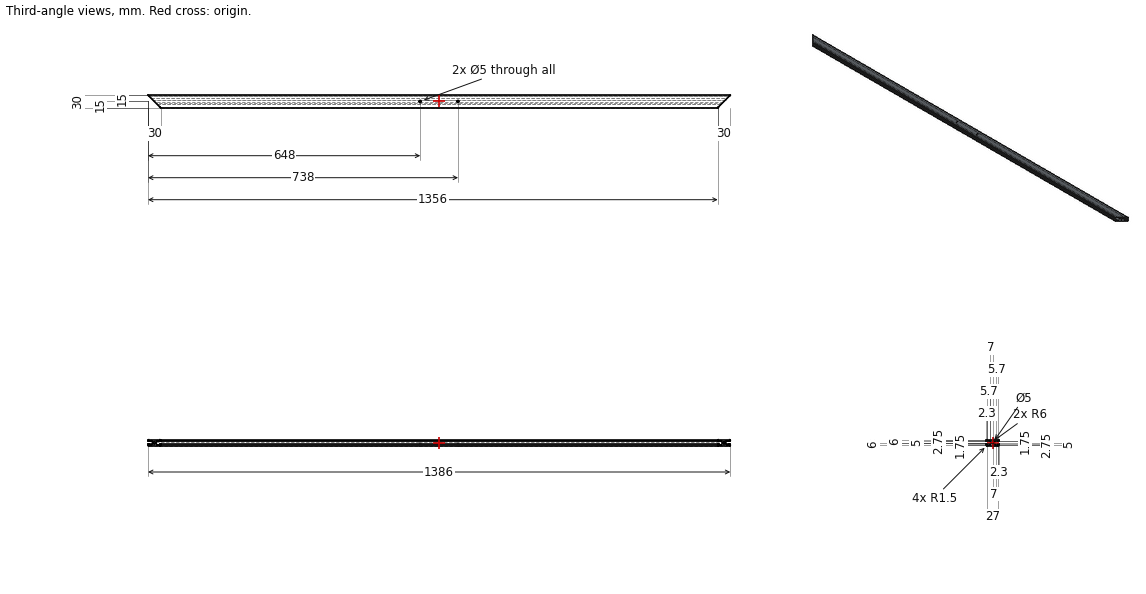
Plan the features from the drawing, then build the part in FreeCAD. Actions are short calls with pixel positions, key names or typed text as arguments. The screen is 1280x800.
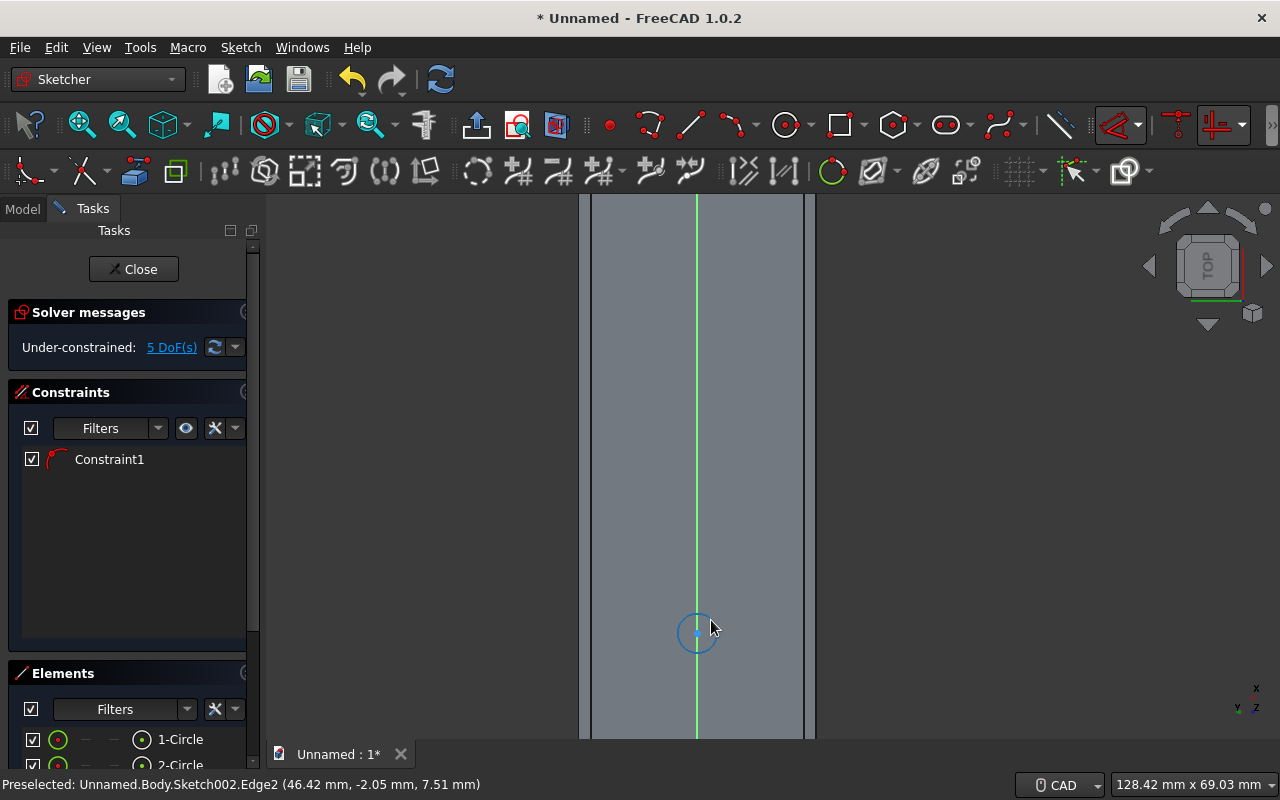
click(711, 619)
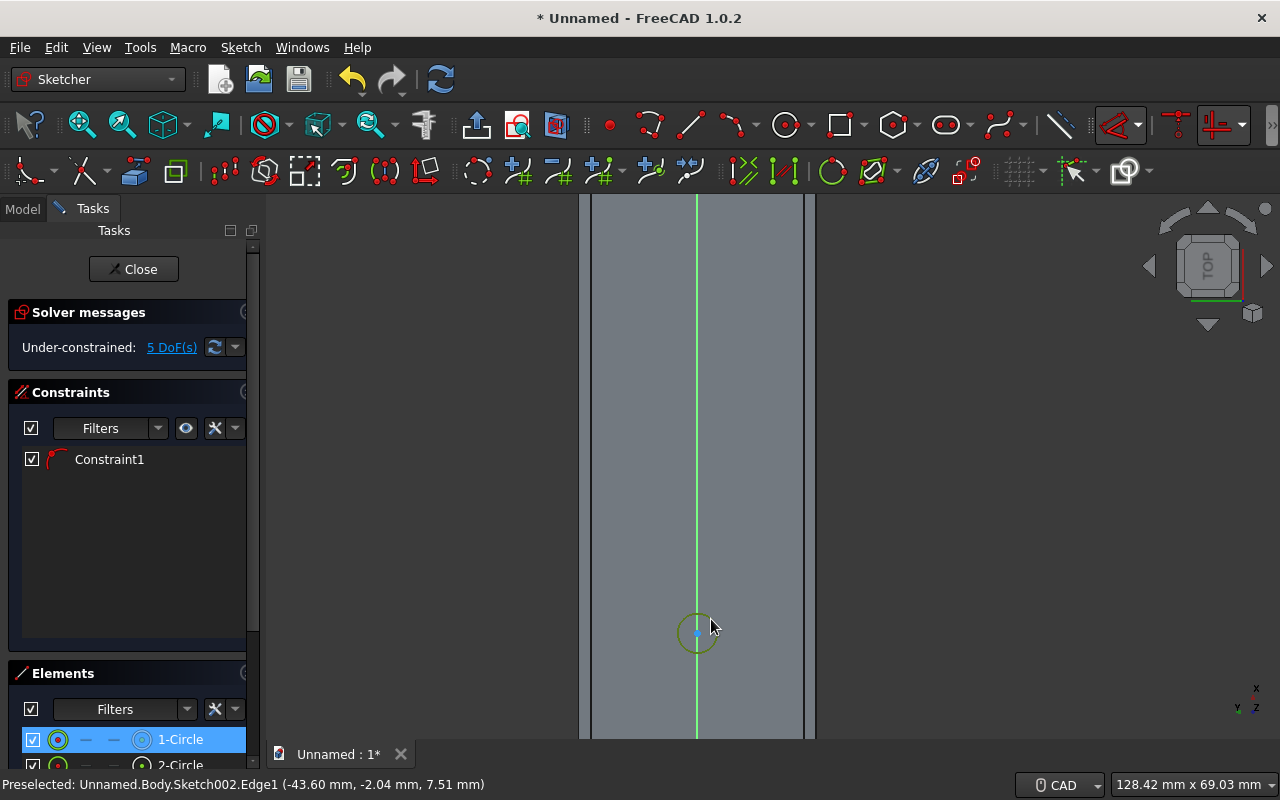
scroll(710, 621, down, 4)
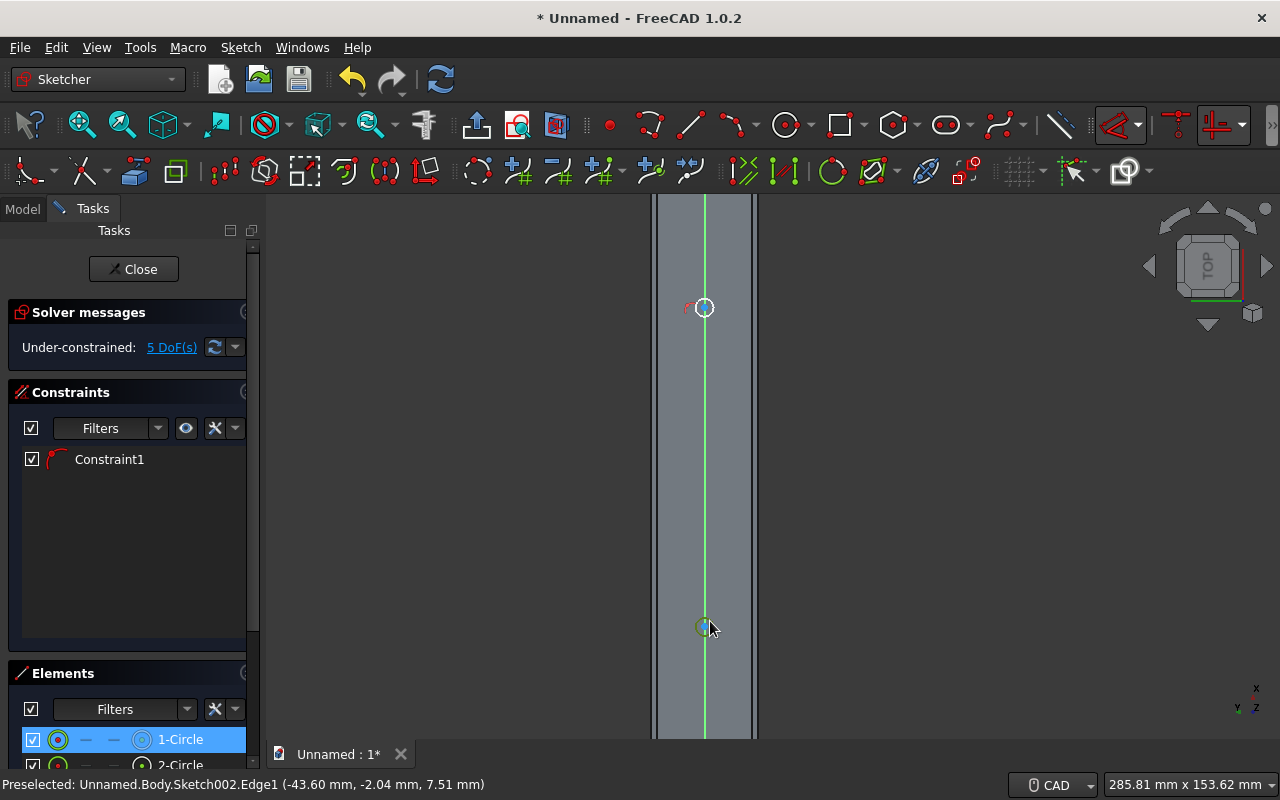
scroll(711, 301, up, 4)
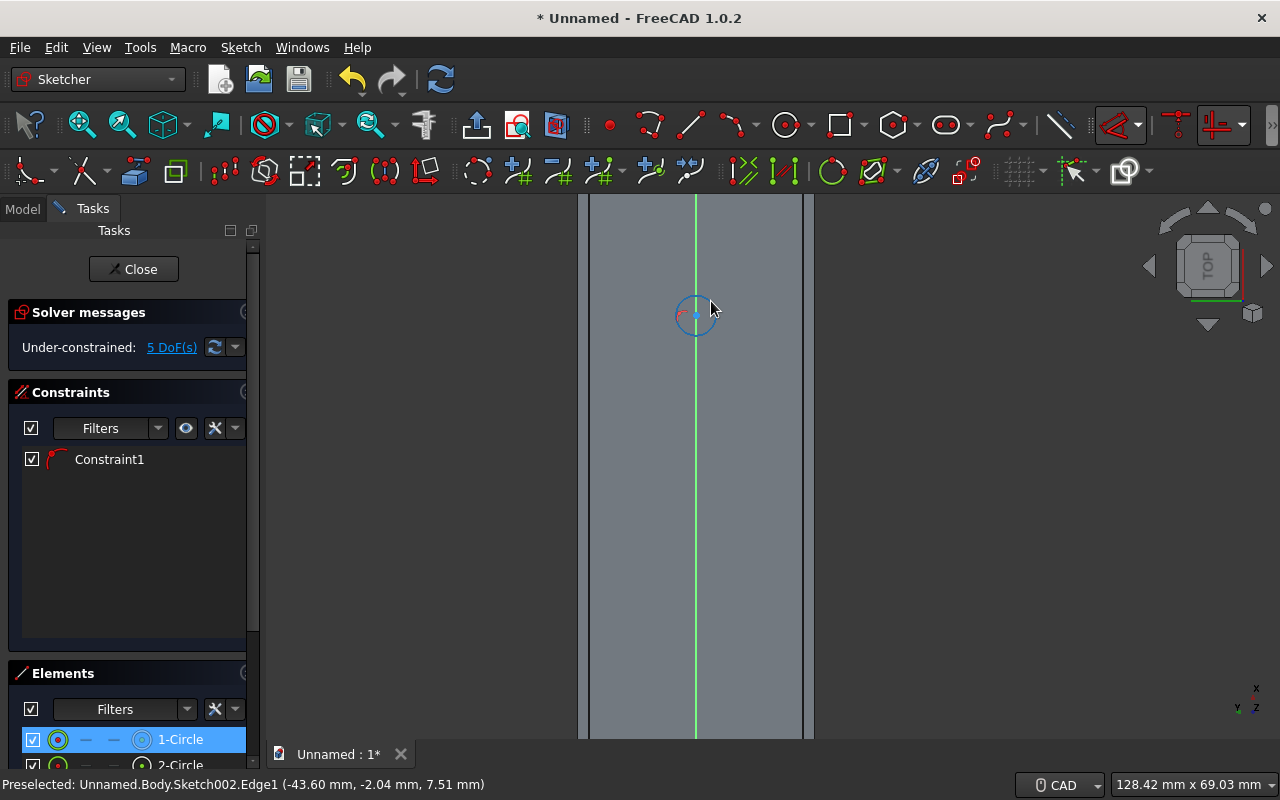
click(710, 301)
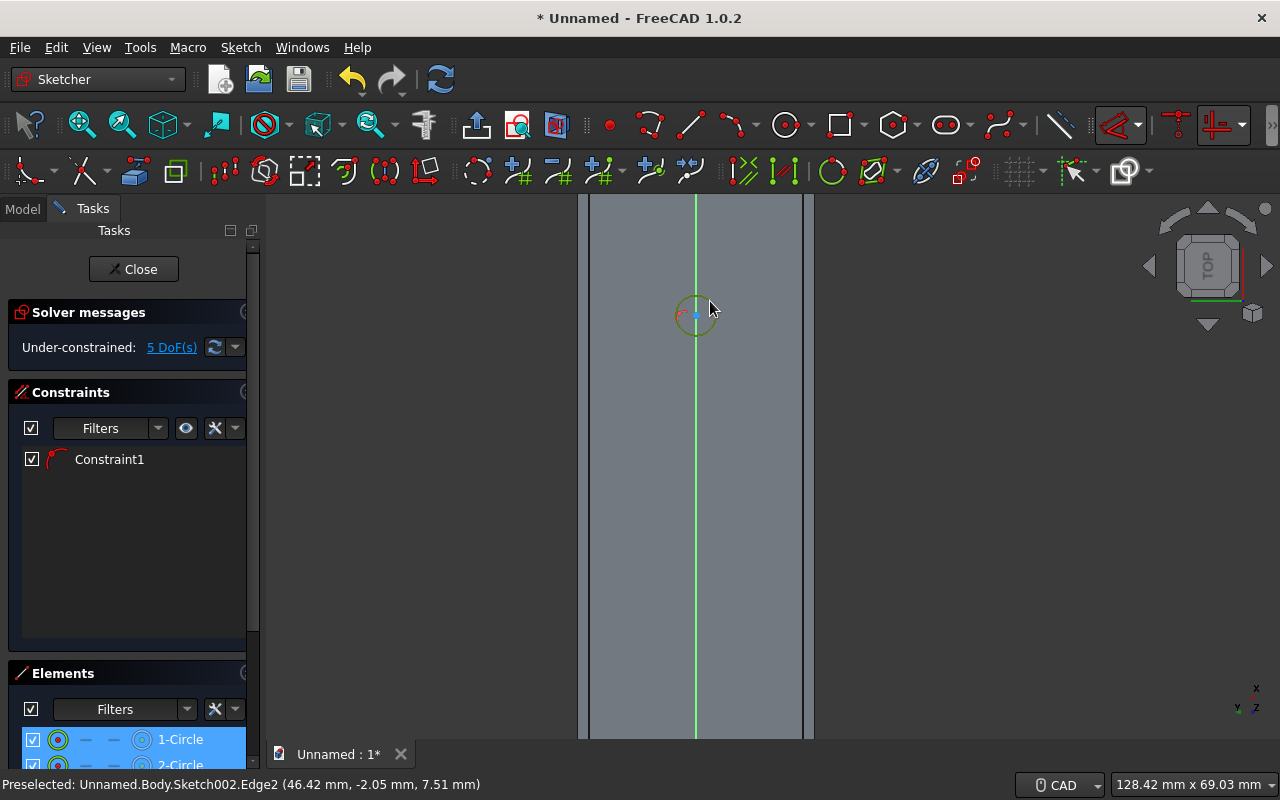
key(e)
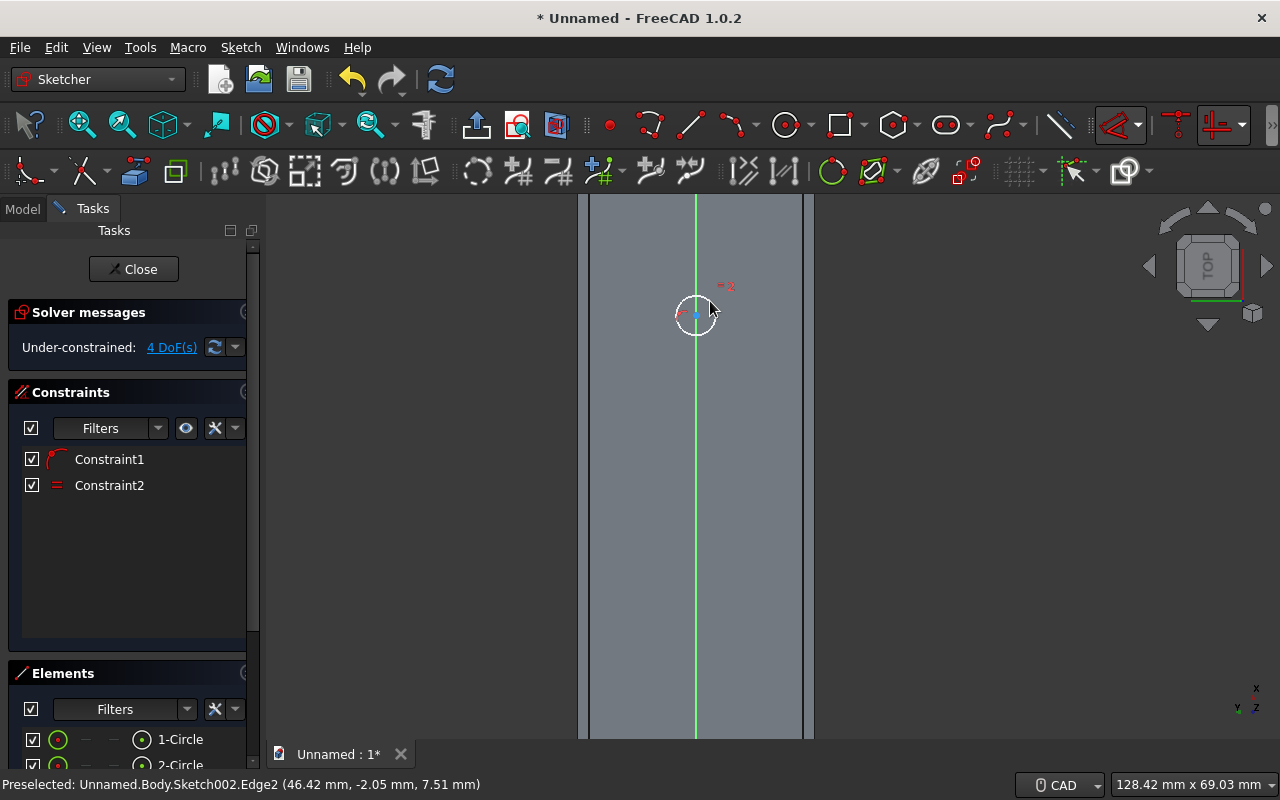
scroll(711, 300, down, 4)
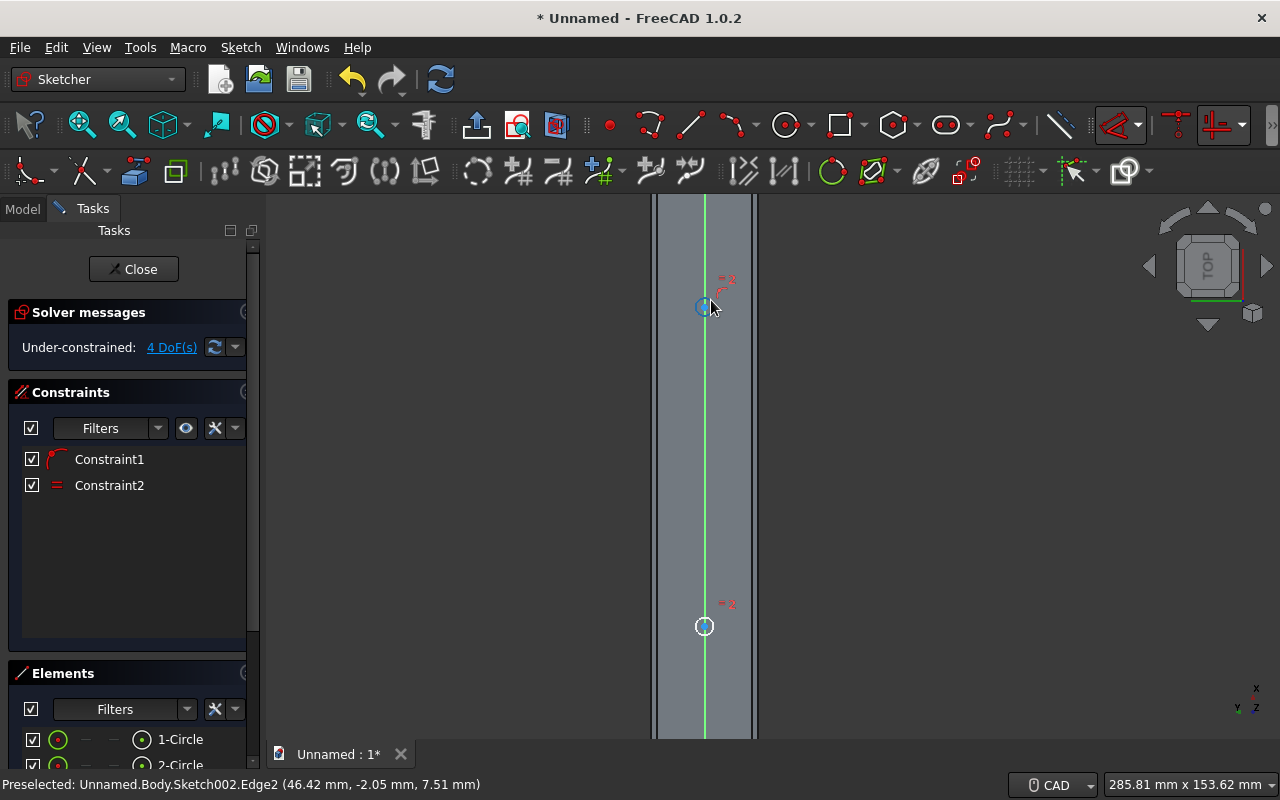
click(705, 626)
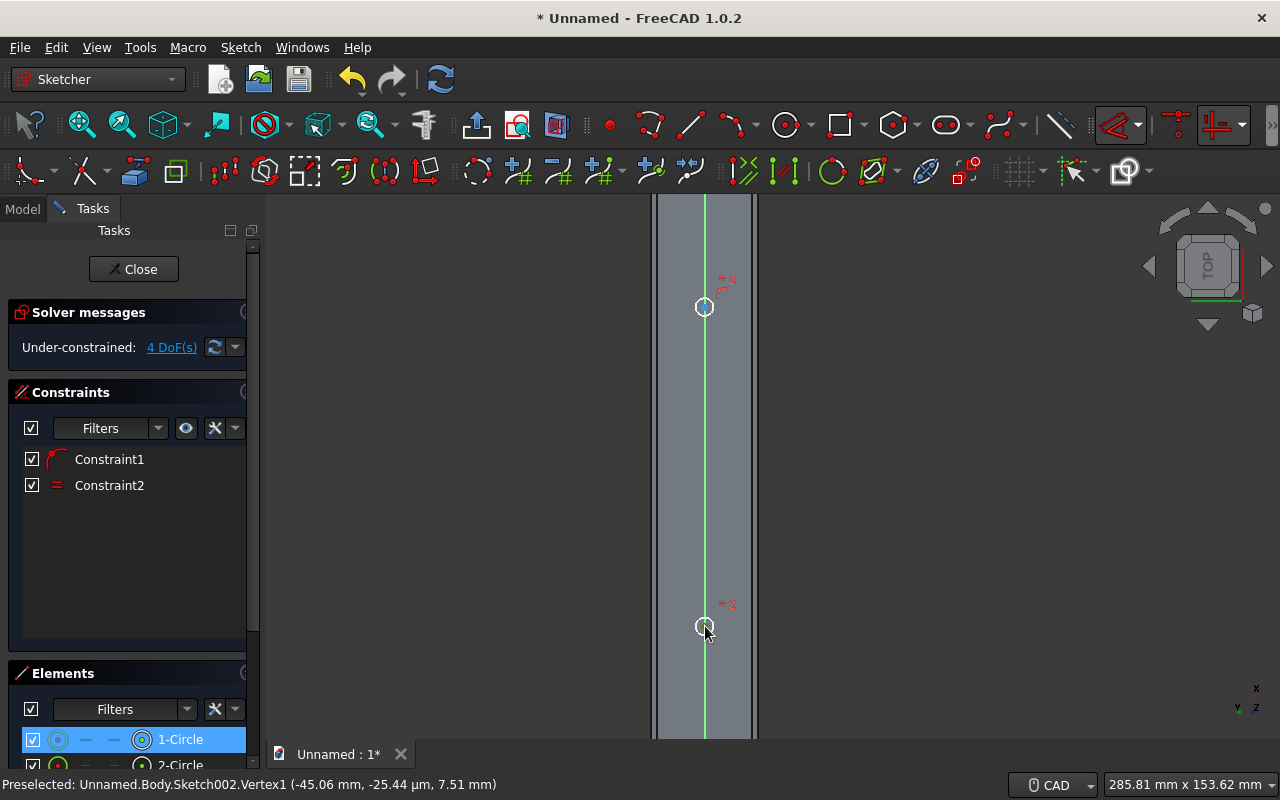
click(705, 676)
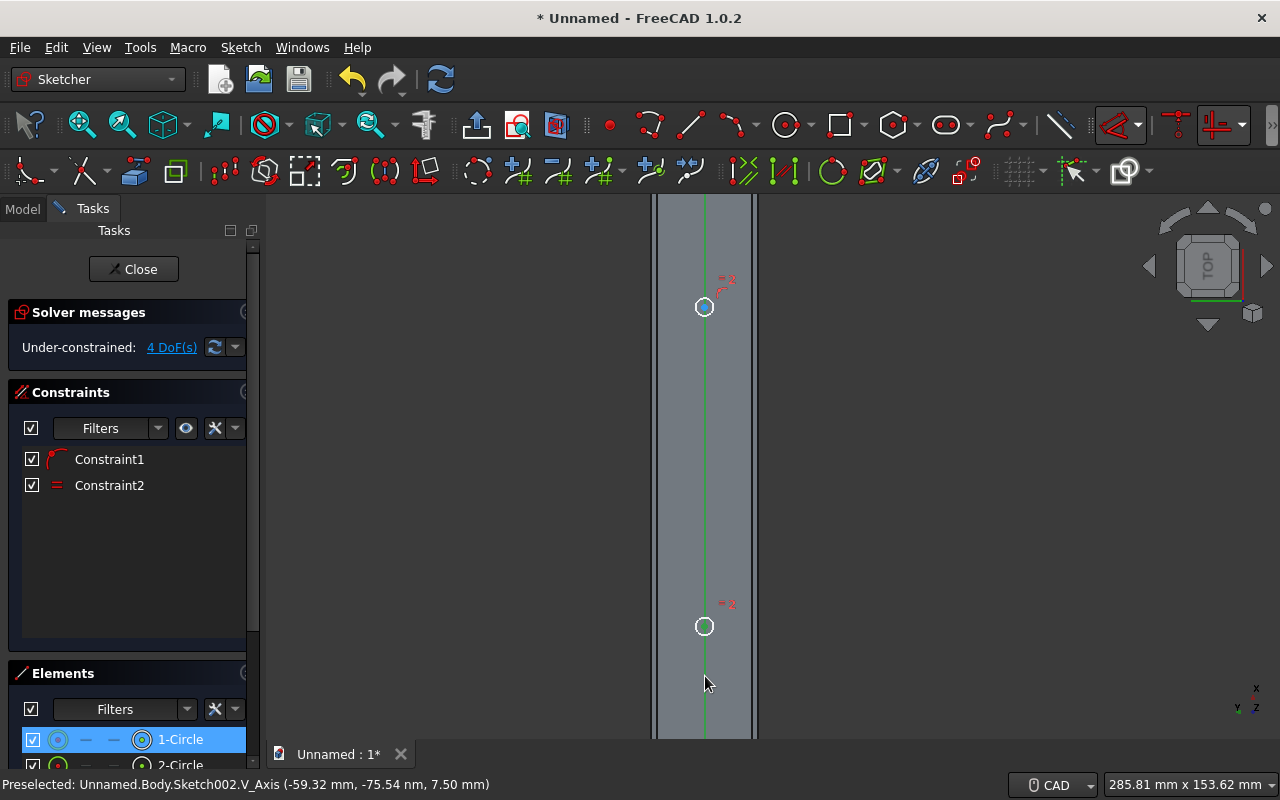
click(1176, 126)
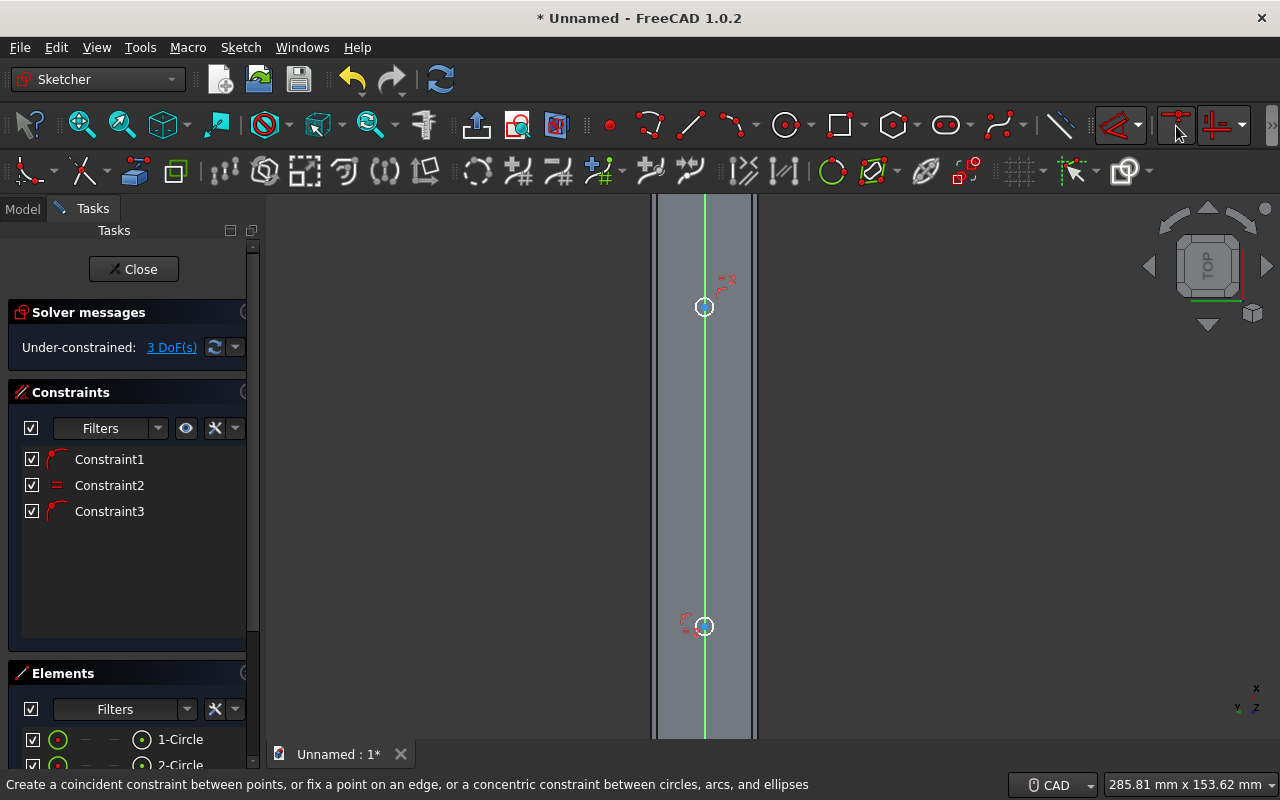
scroll(705, 618, up, 5)